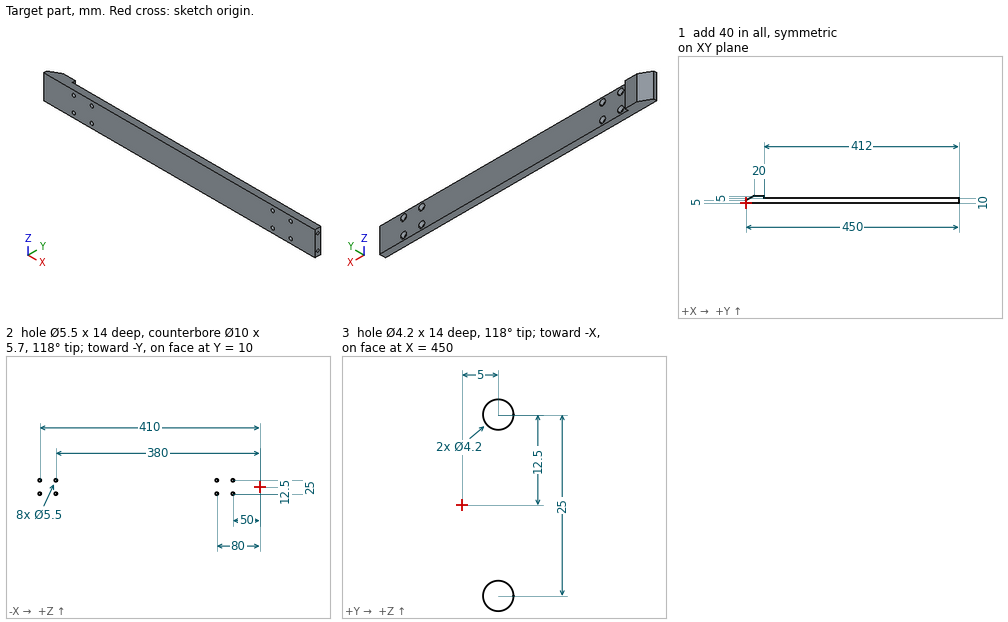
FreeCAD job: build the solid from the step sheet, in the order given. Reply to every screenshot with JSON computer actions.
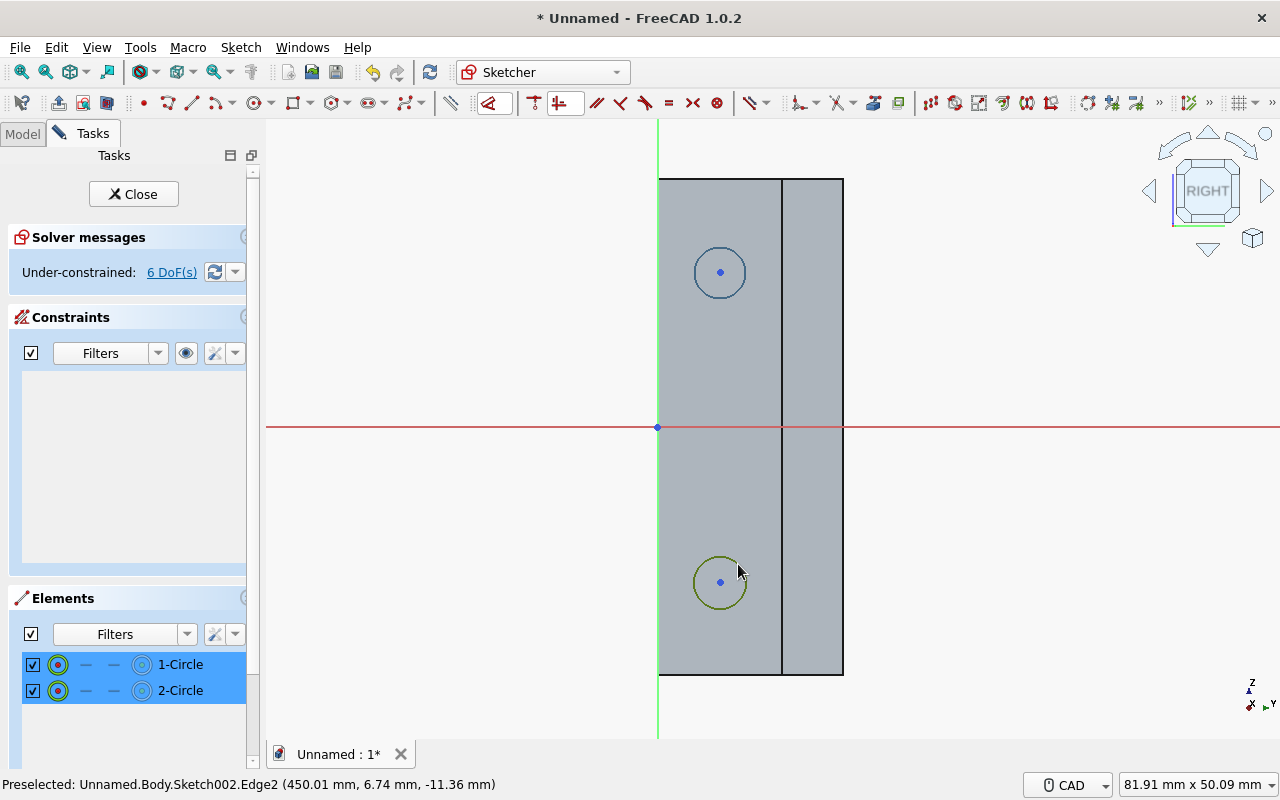
{"action": "left_click", "coordinate": [670, 104]}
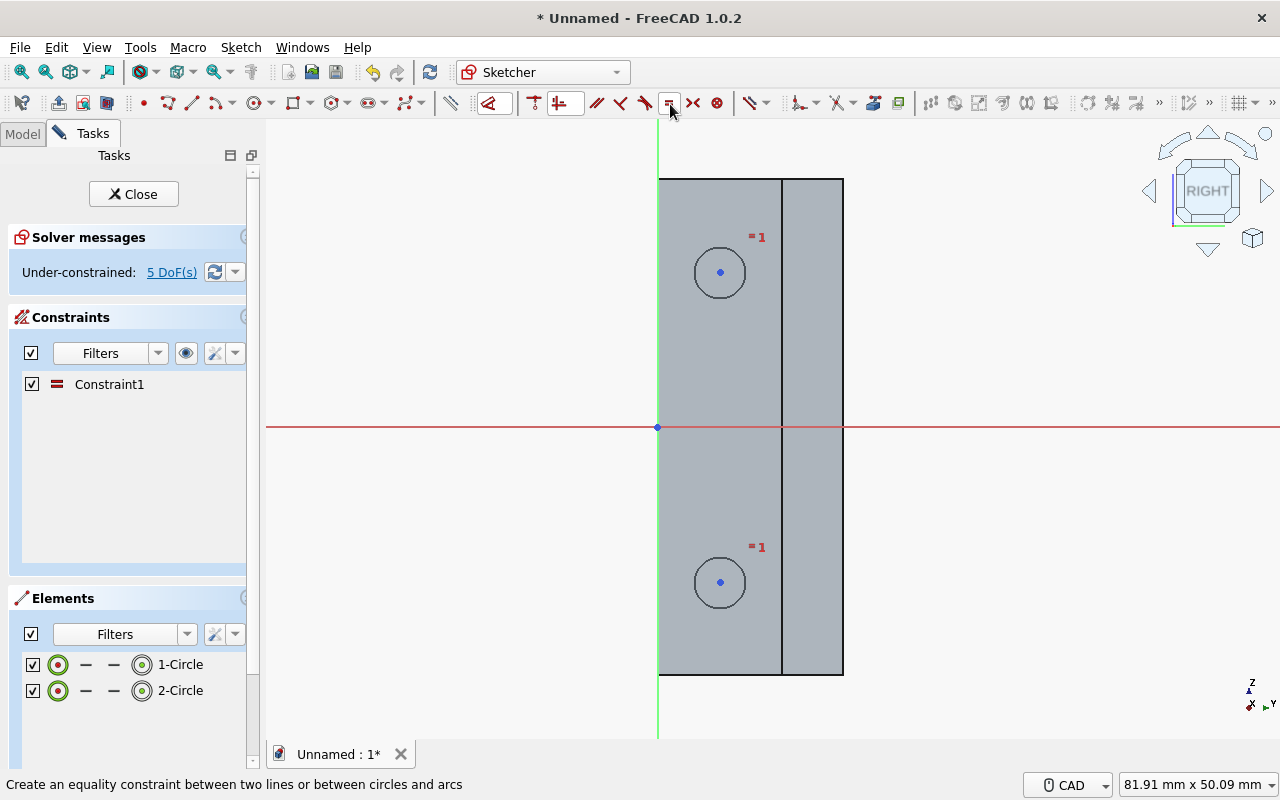
{"action": "left_click", "coordinate": [720, 273]}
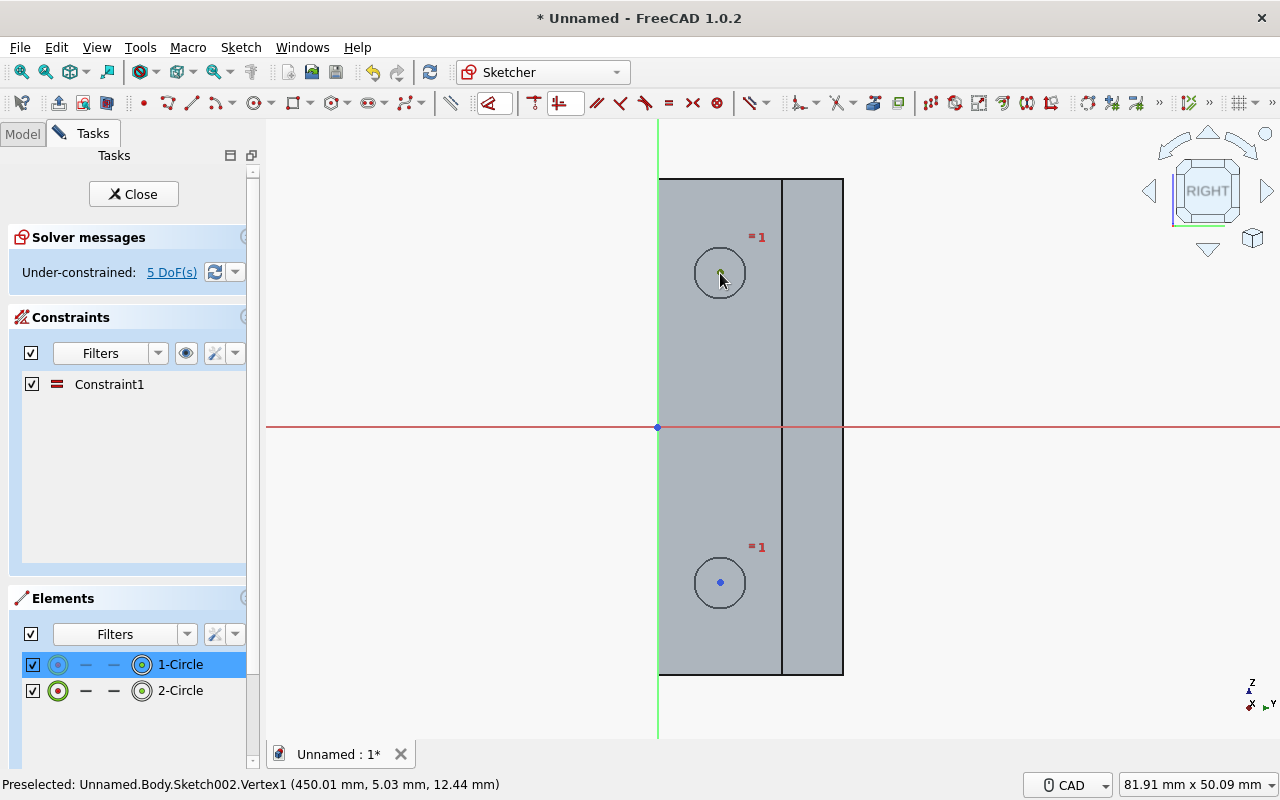
{"action": "left_click", "coordinate": [720, 583]}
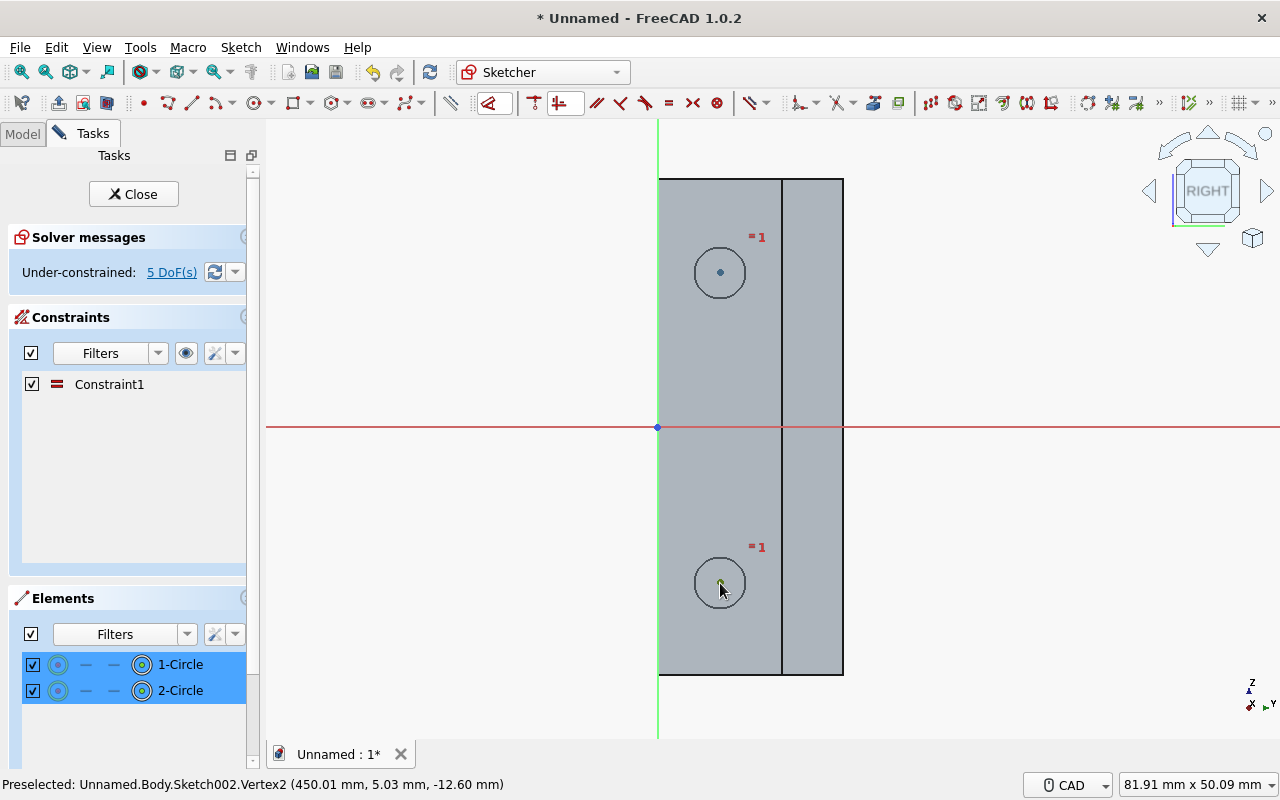
{"action": "key", "text": "v"}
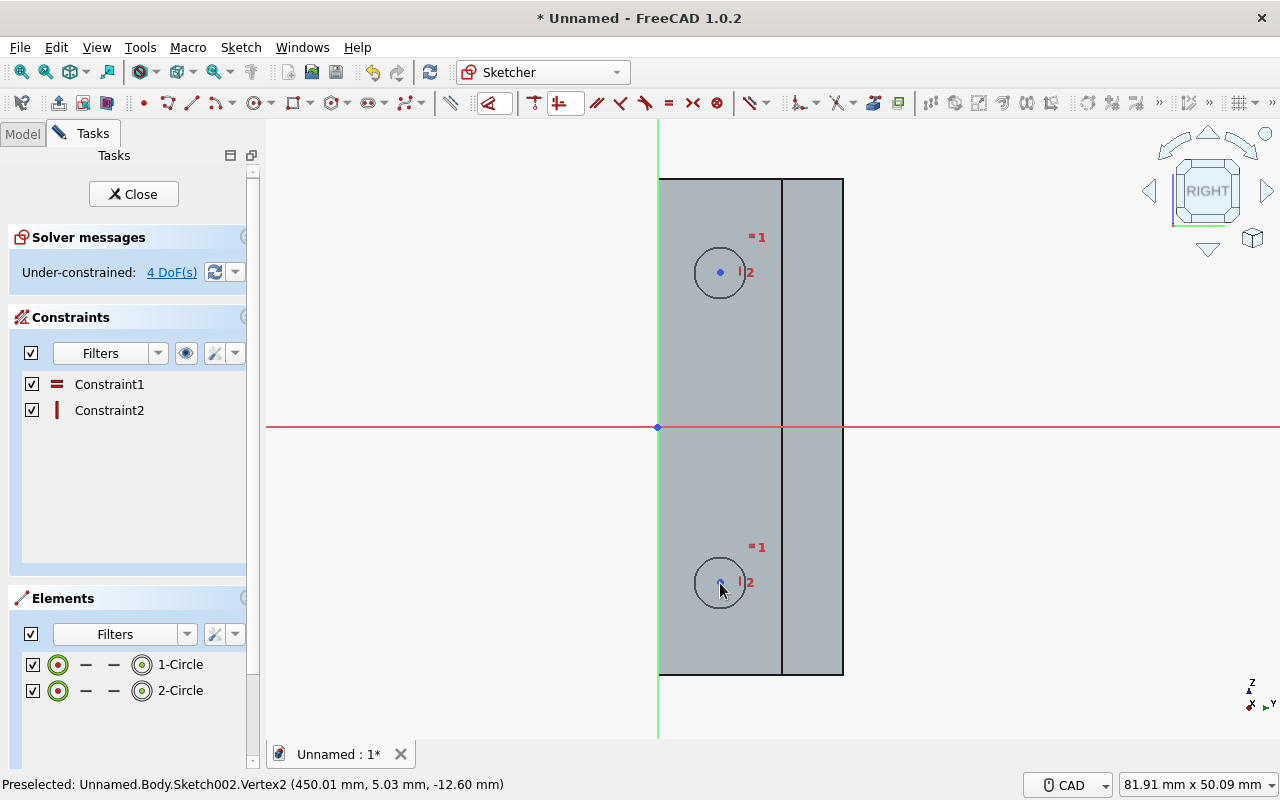
{"action": "left_click", "coordinate": [738, 255]}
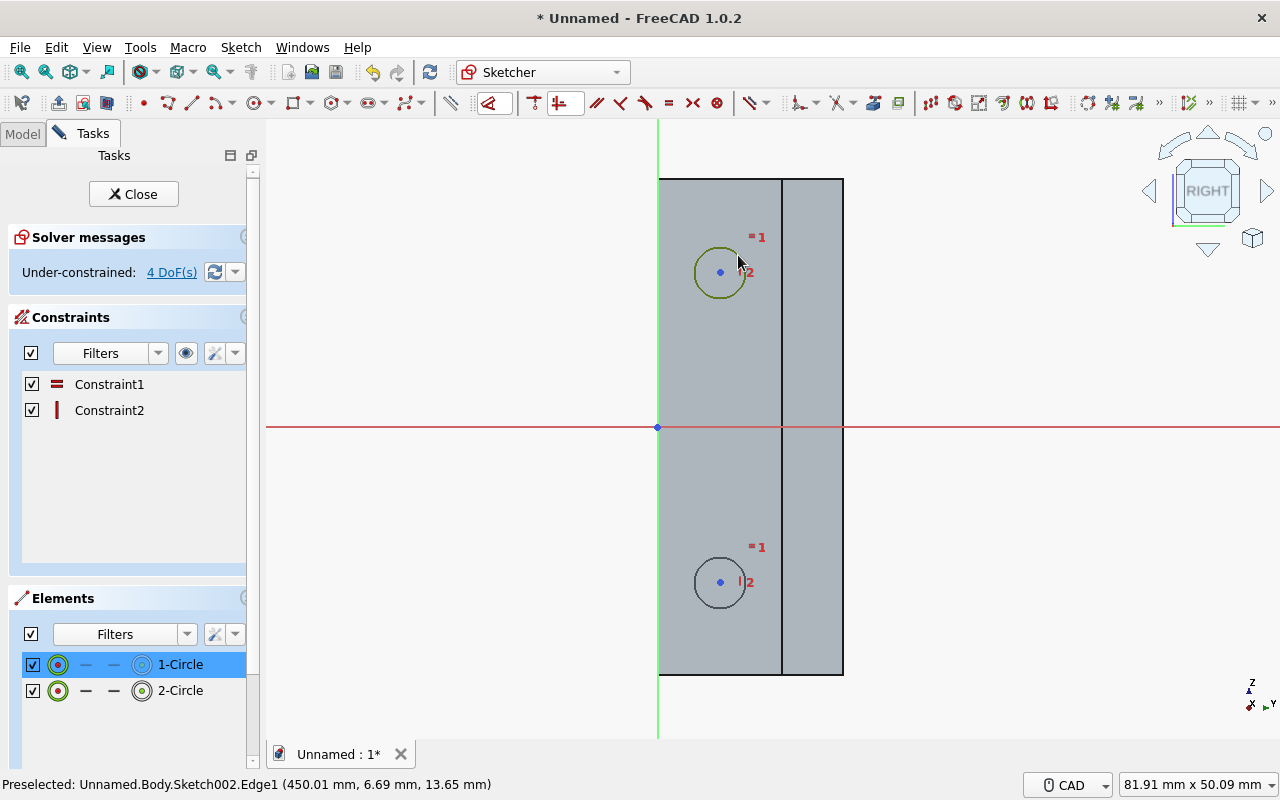
{"action": "key", "text": "k o"}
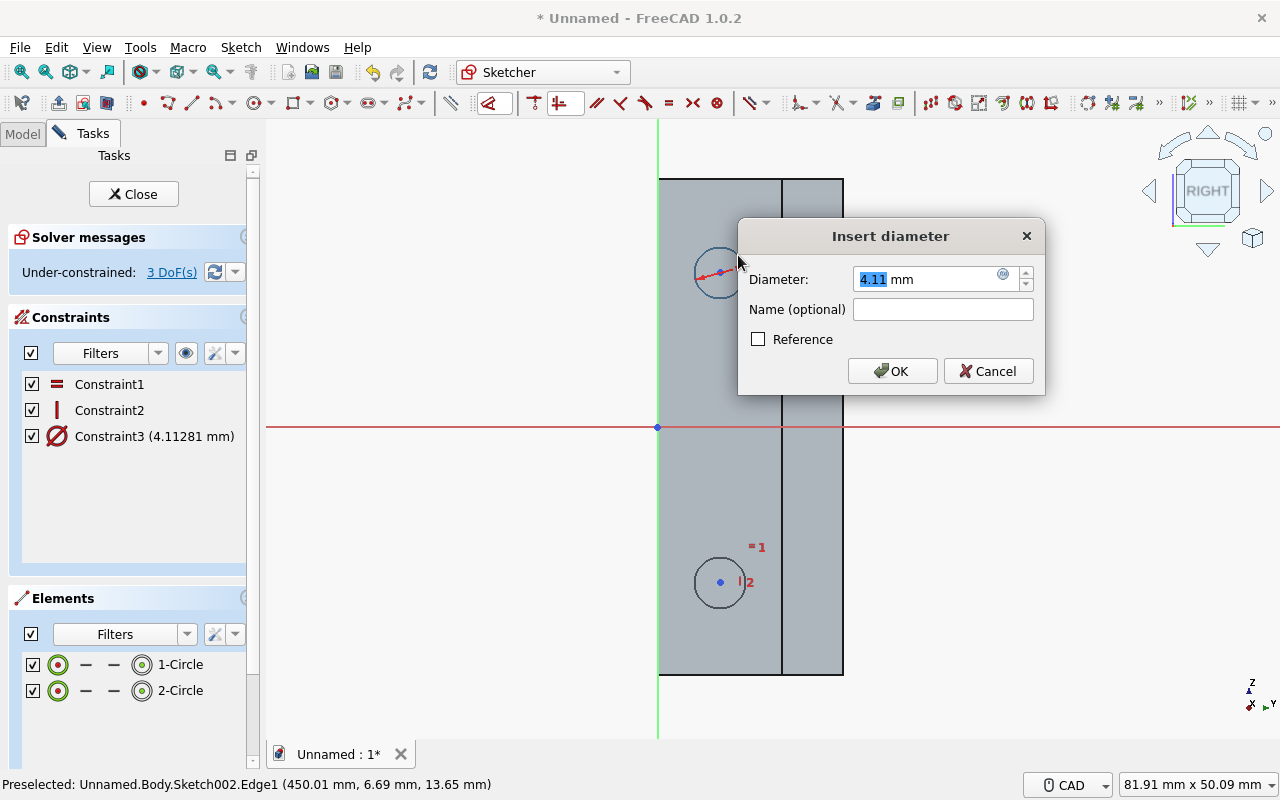
{"action": "type", "text": "4.2"}
{"action": "key", "text": "Return"}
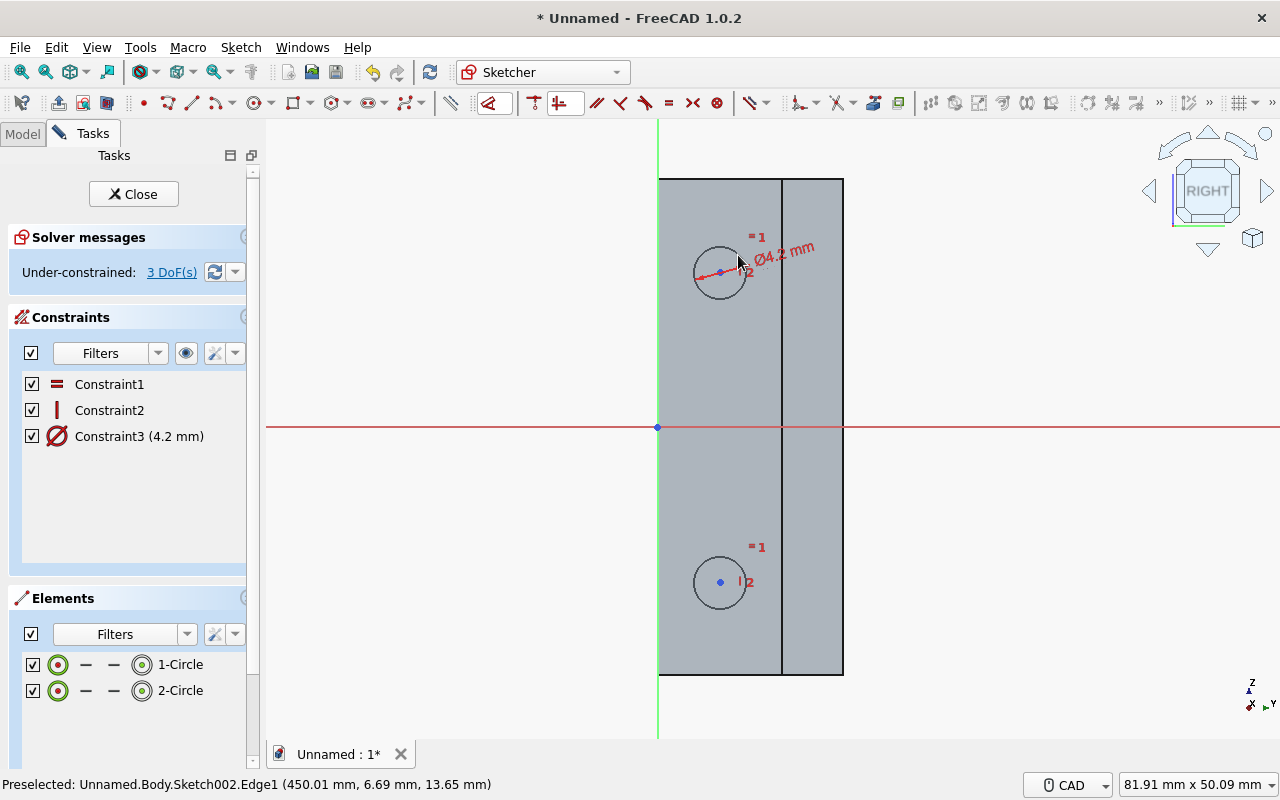
{"action": "left_click", "coordinate": [720, 273]}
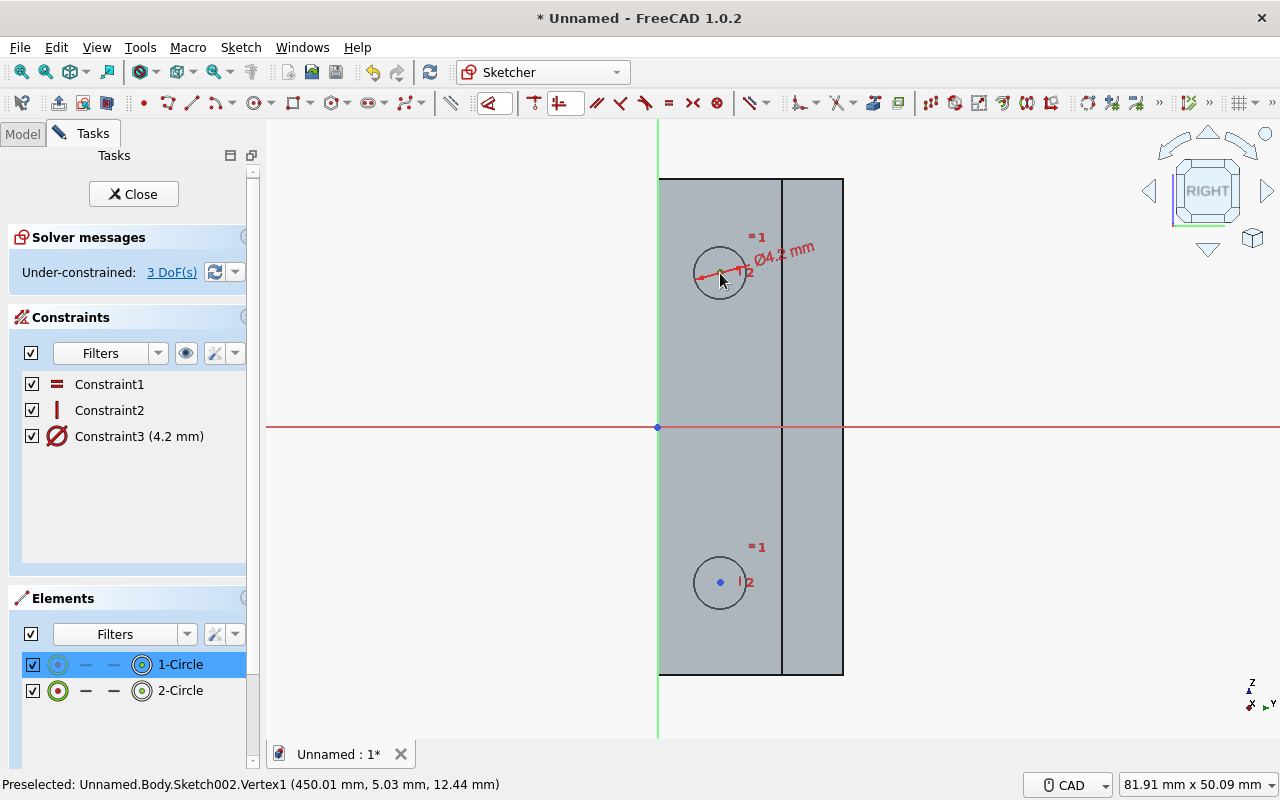
{"action": "key", "text": "l"}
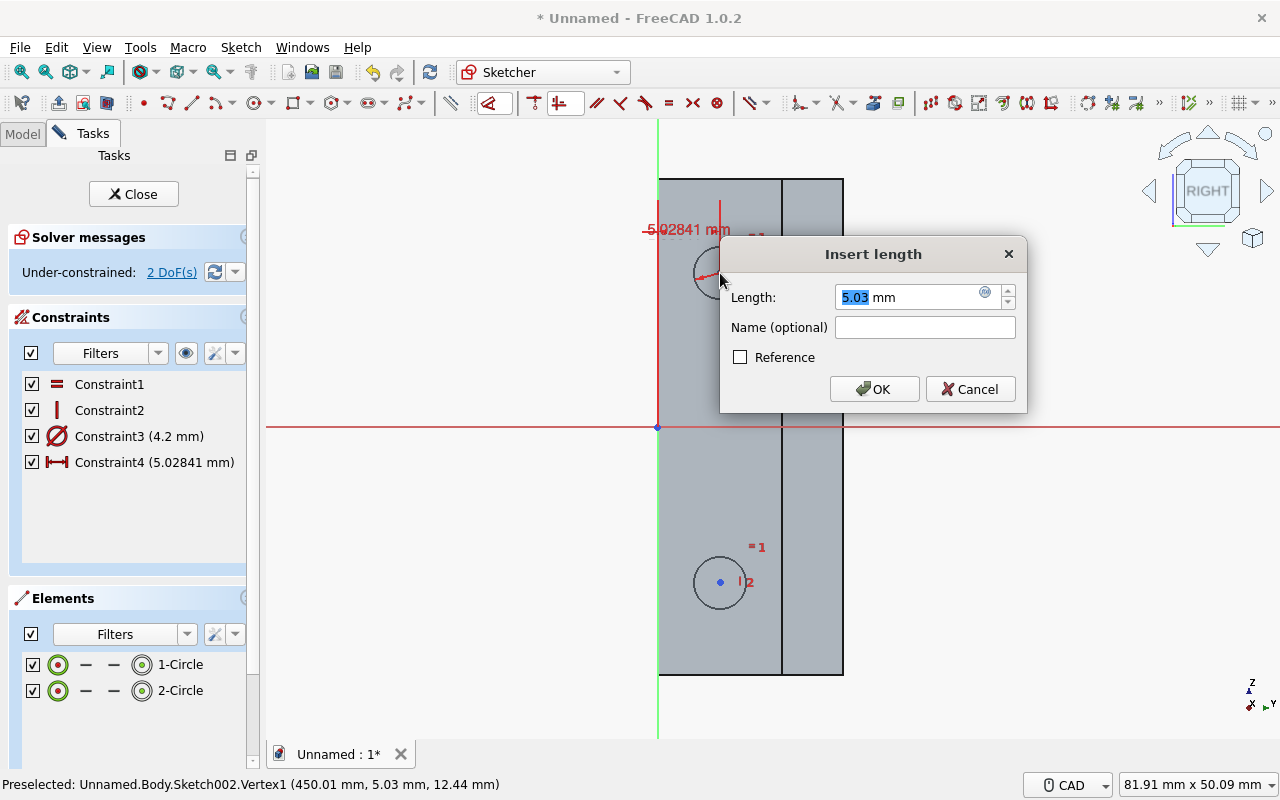
{"action": "type", "text": "5"}
{"action": "key", "text": "Return"}